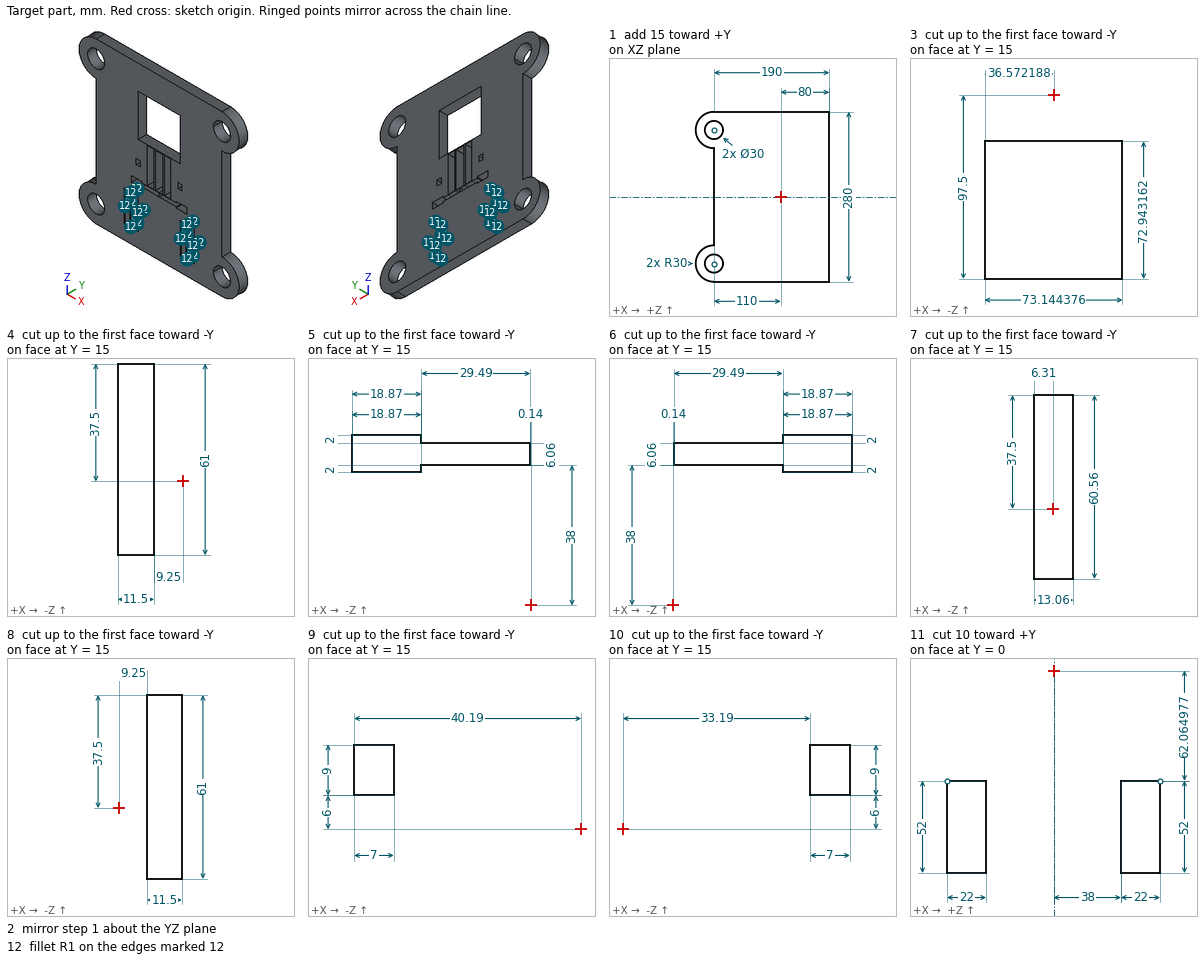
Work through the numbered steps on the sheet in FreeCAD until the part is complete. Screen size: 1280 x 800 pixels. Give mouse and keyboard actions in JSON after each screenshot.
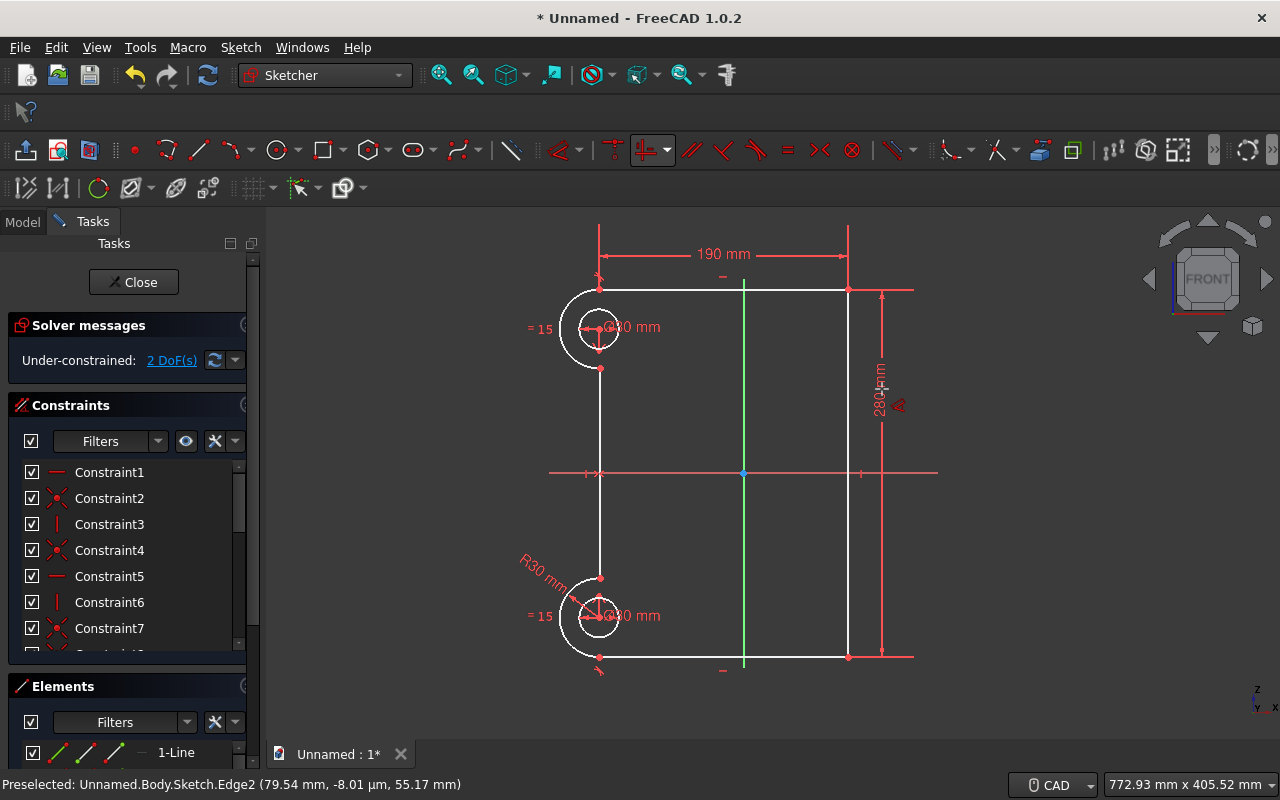
{"action": "left_click", "coordinate": [848, 290]}
{"action": "left_click", "coordinate": [796, 256]}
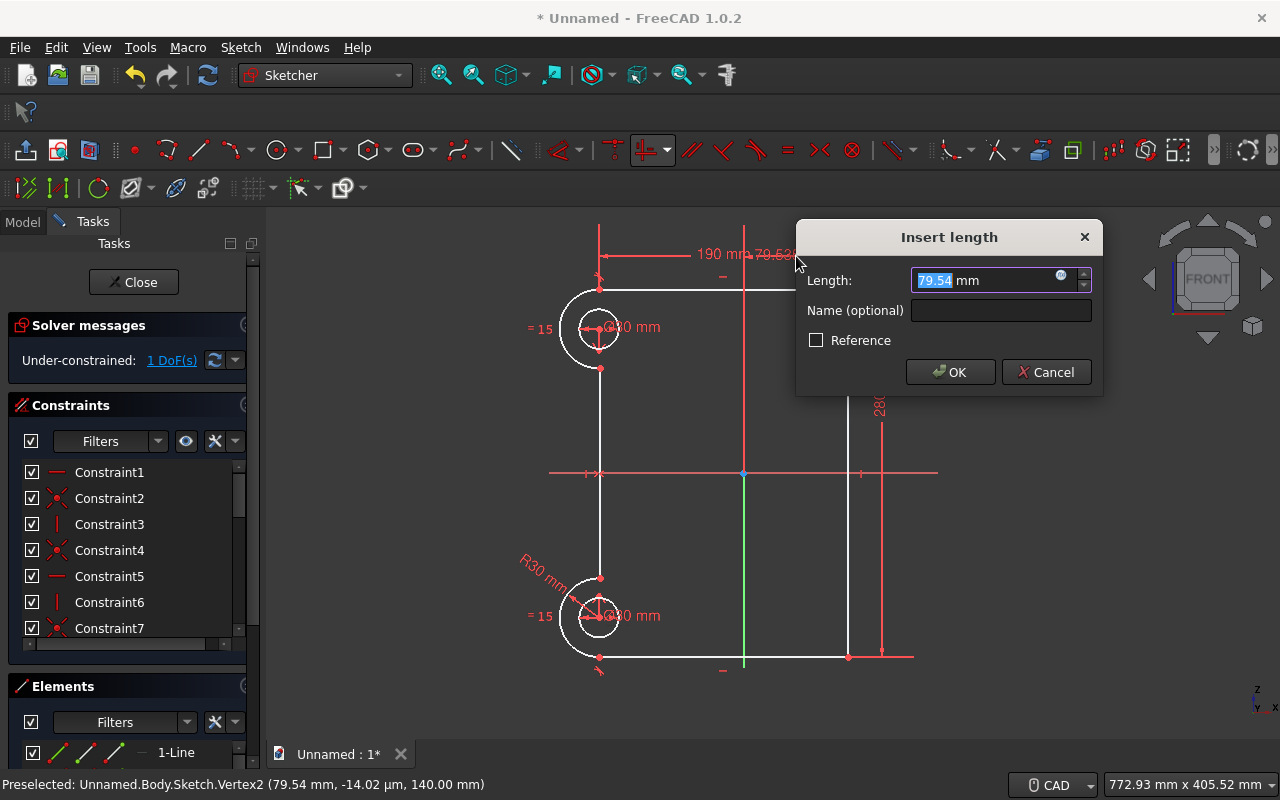
{"action": "type", "text": "80"}
{"action": "key", "text": "Return"}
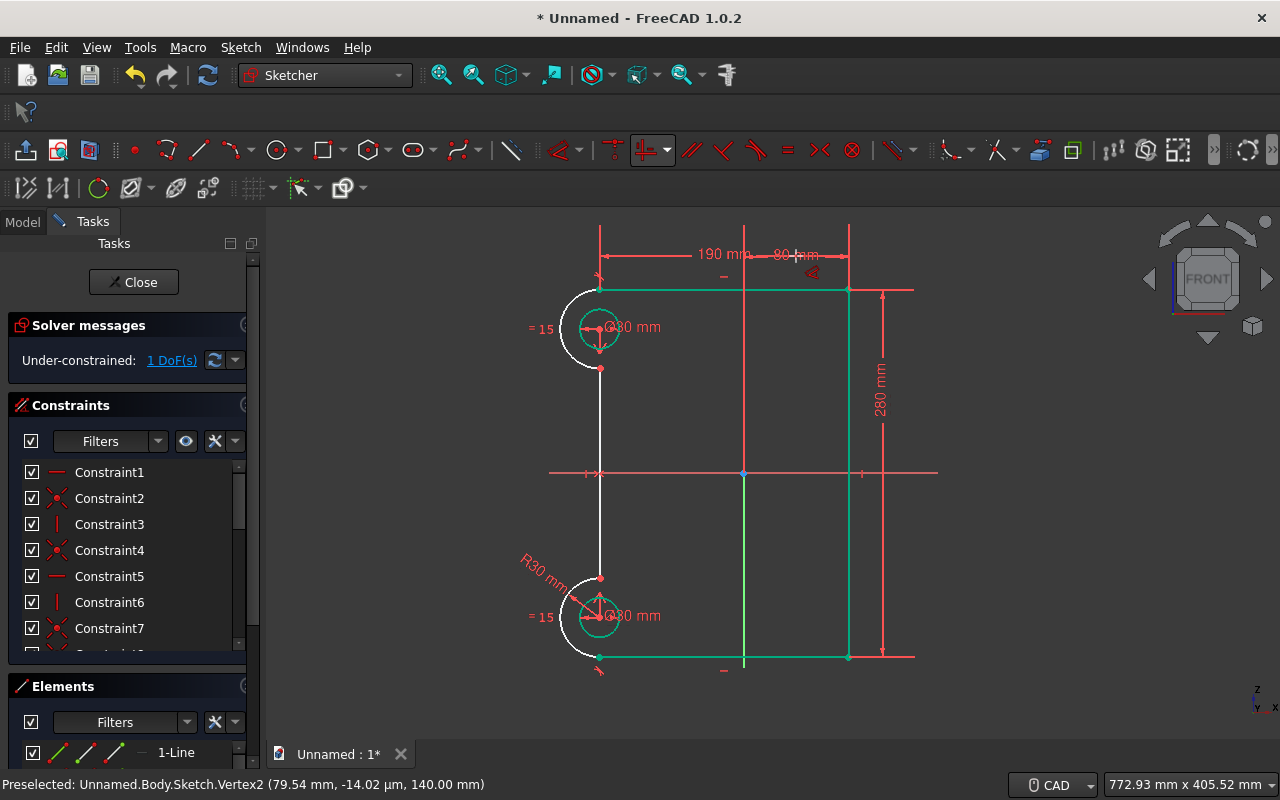
{"action": "left_click", "coordinate": [600, 578]}
{"action": "left_click", "coordinate": [672, 612]}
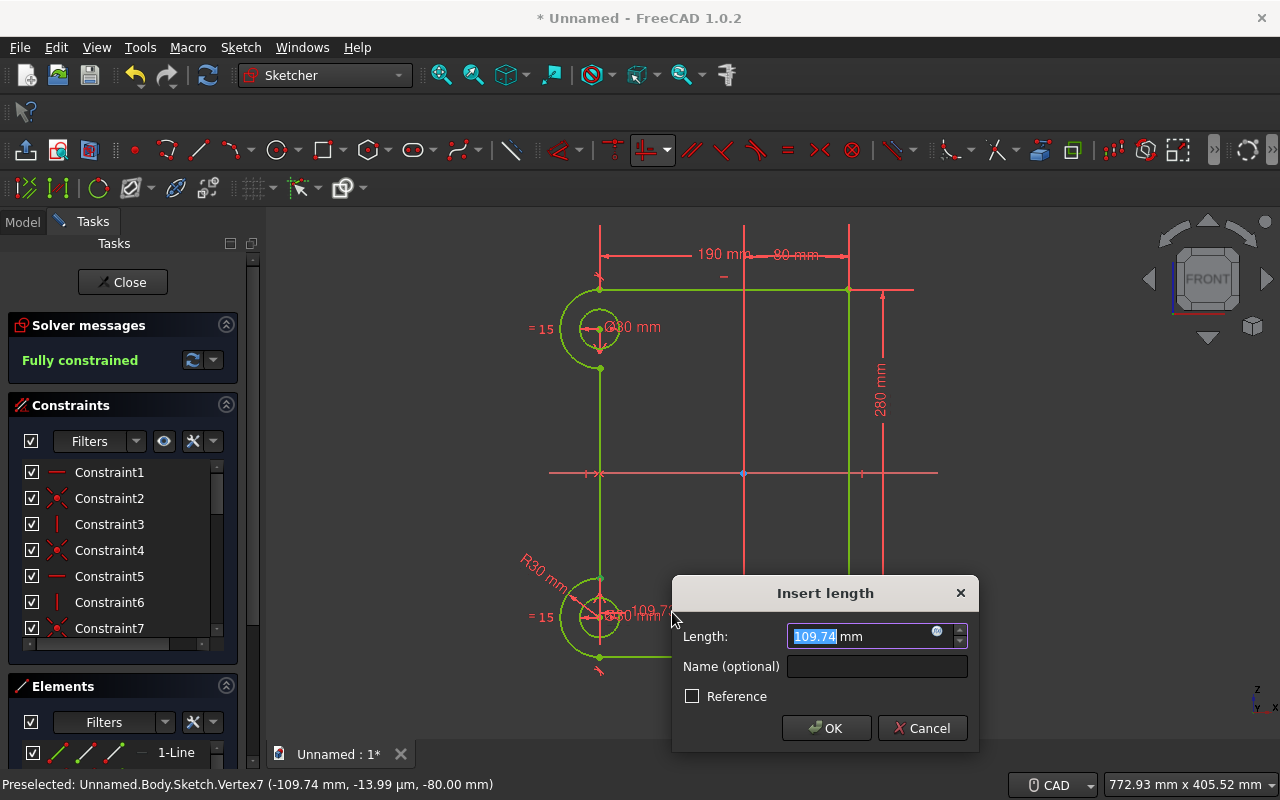
{"action": "type", "text": "110"}
{"action": "key", "text": "Return"}
{"action": "key", "text": "Escape"}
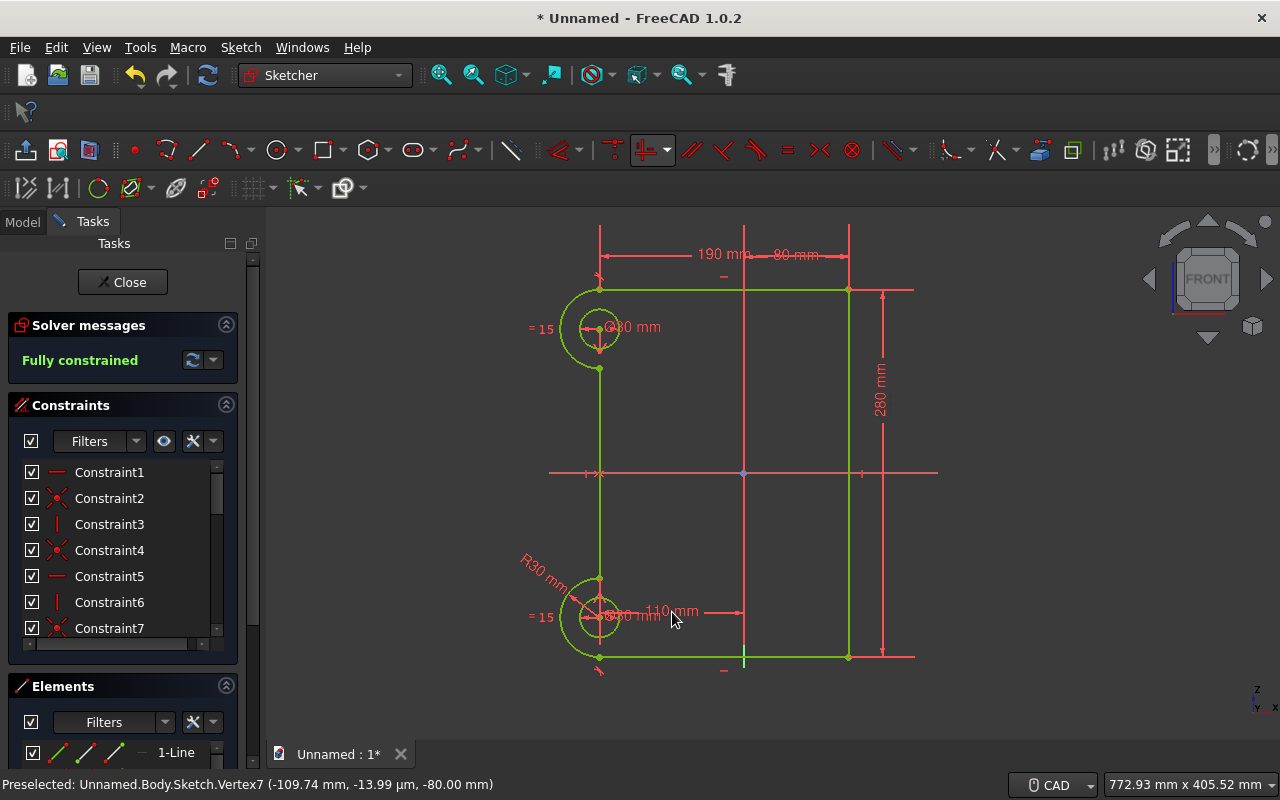
{"action": "left_click", "coordinate": [123, 282]}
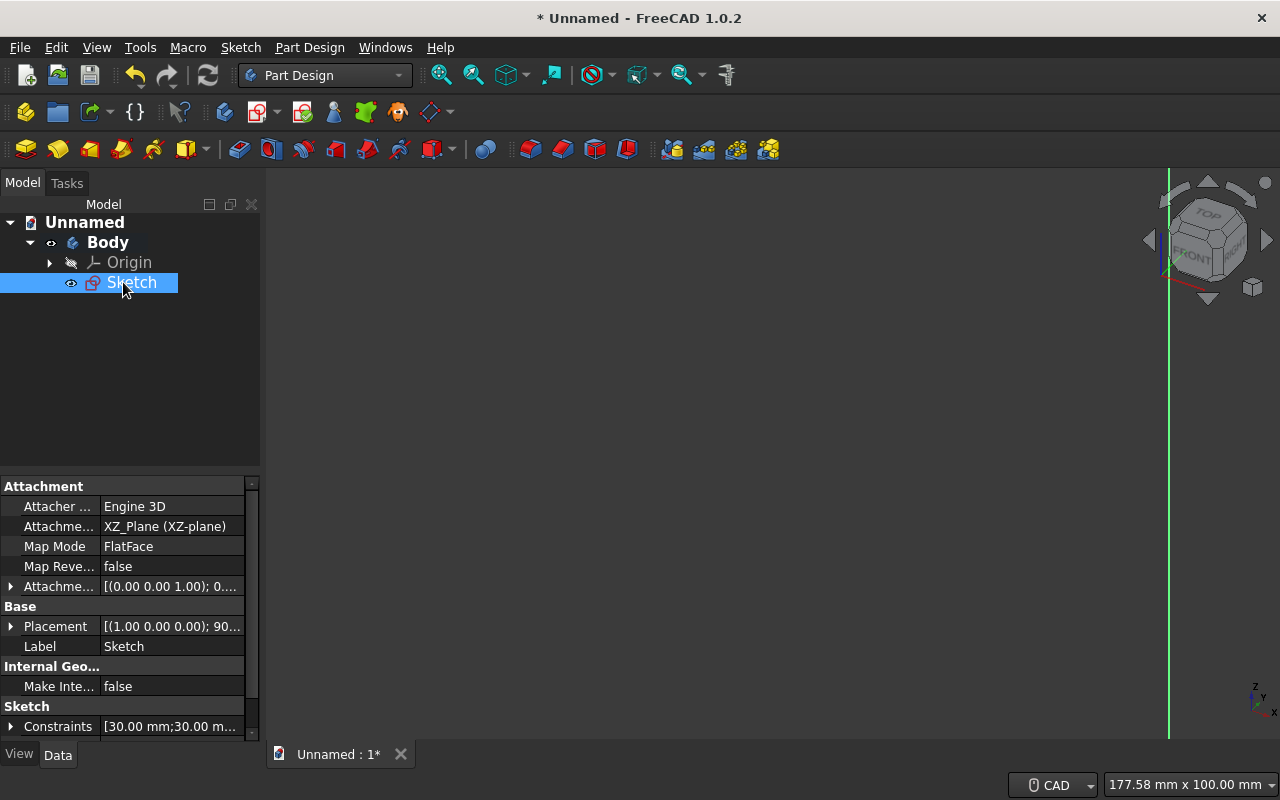
{"action": "left_click", "coordinate": [26, 150]}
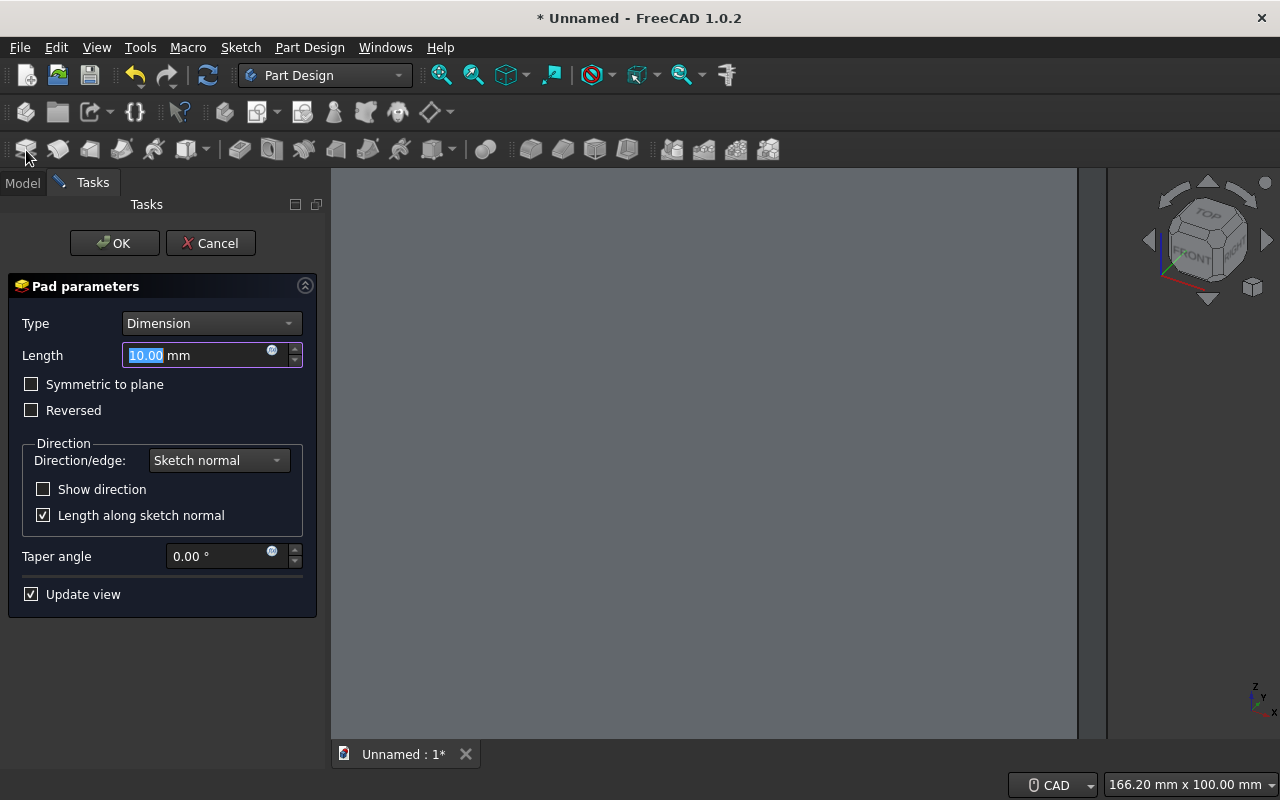
{"action": "type", "text": "15"}
{"action": "key", "text": "Tab"}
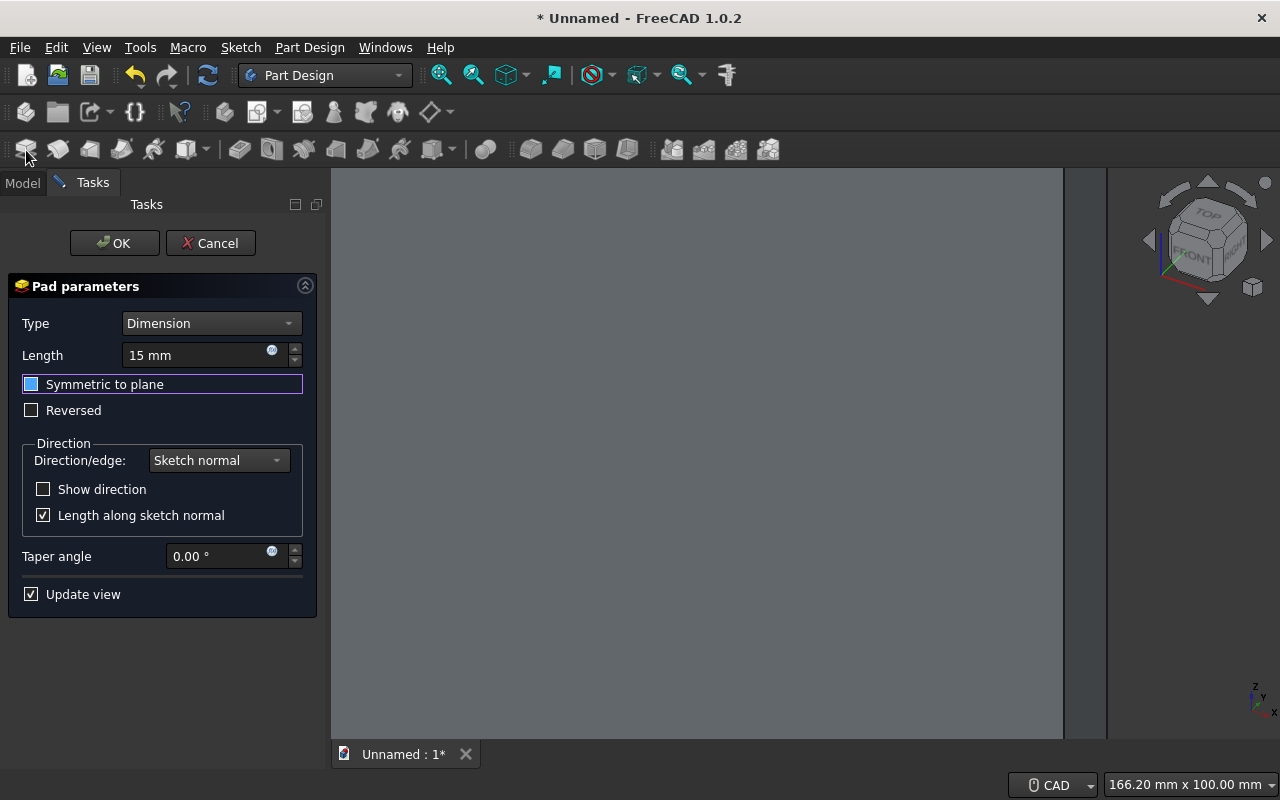
{"action": "left_click", "coordinate": [30, 410]}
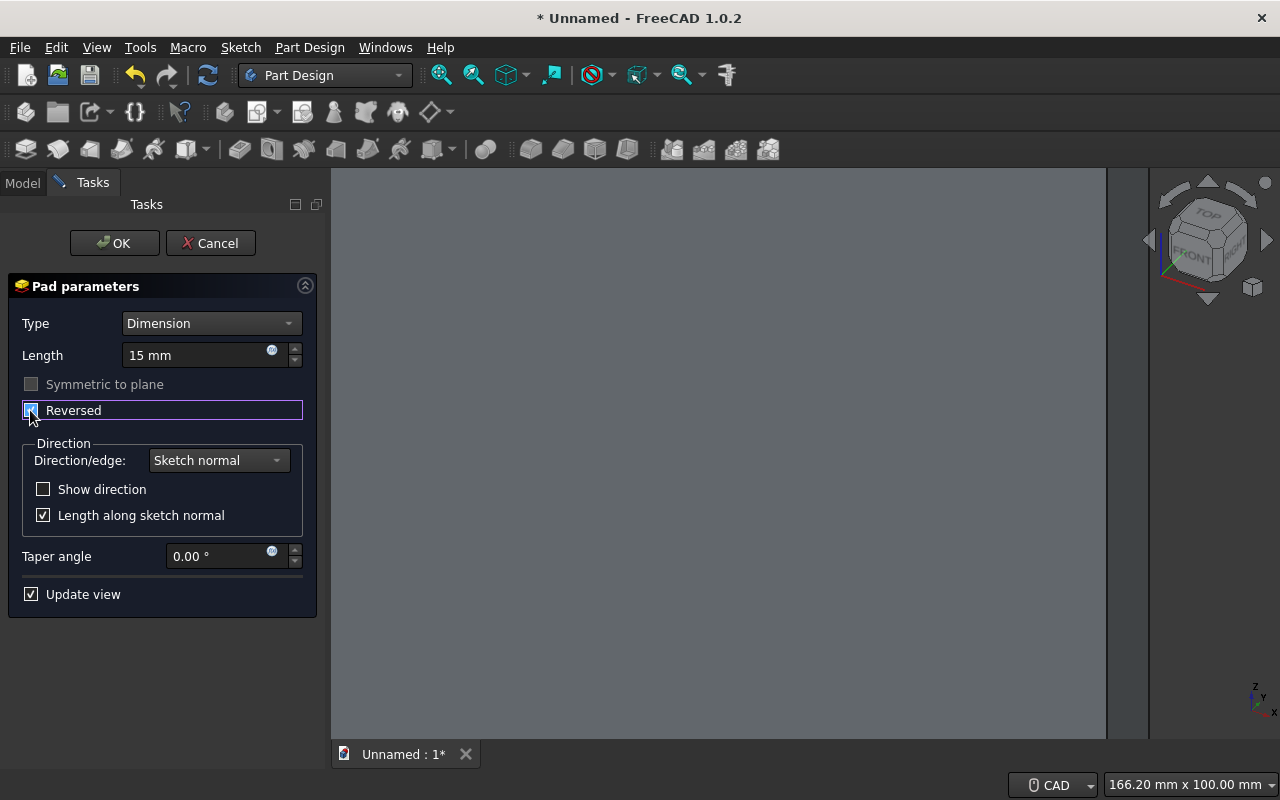
{"action": "left_click", "coordinate": [115, 243]}